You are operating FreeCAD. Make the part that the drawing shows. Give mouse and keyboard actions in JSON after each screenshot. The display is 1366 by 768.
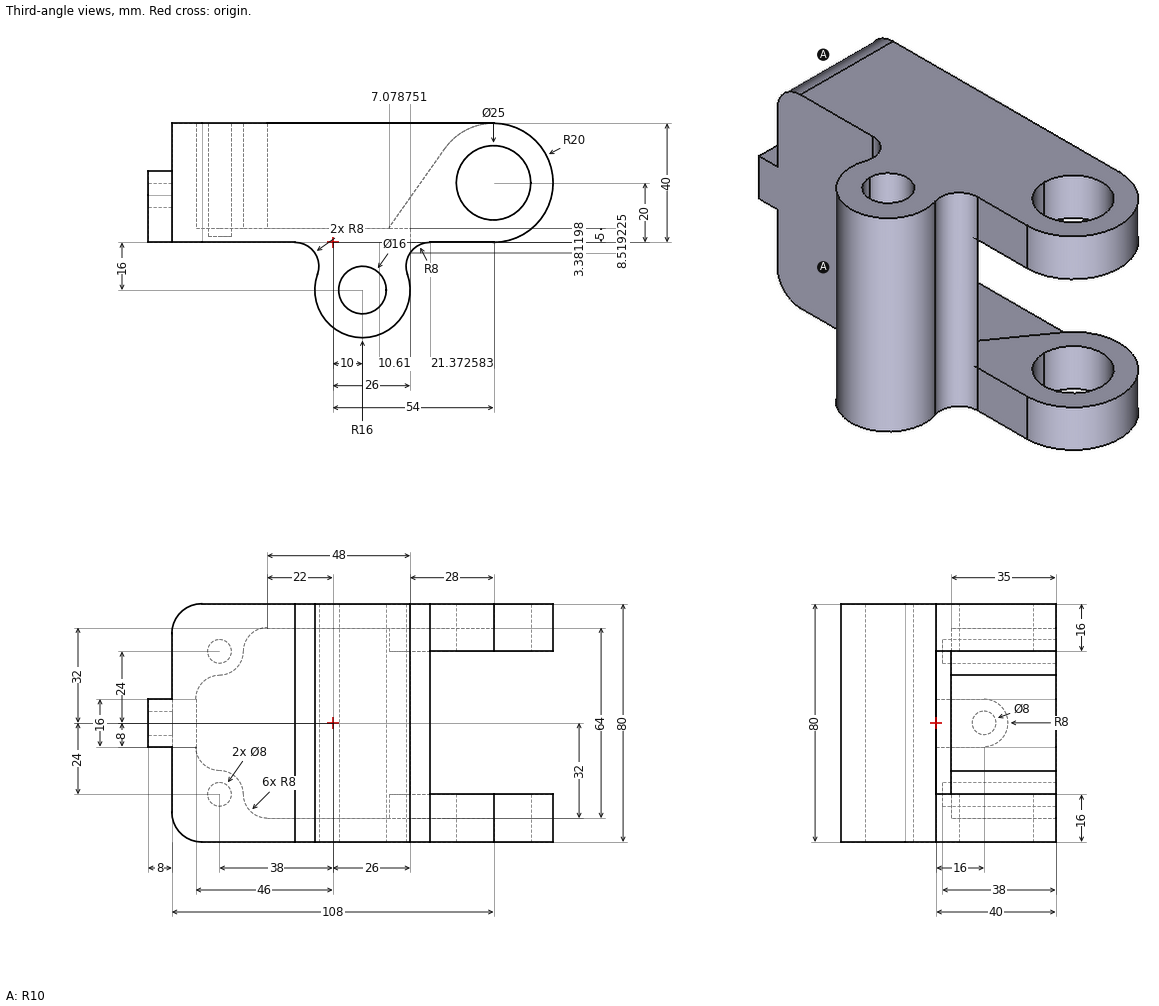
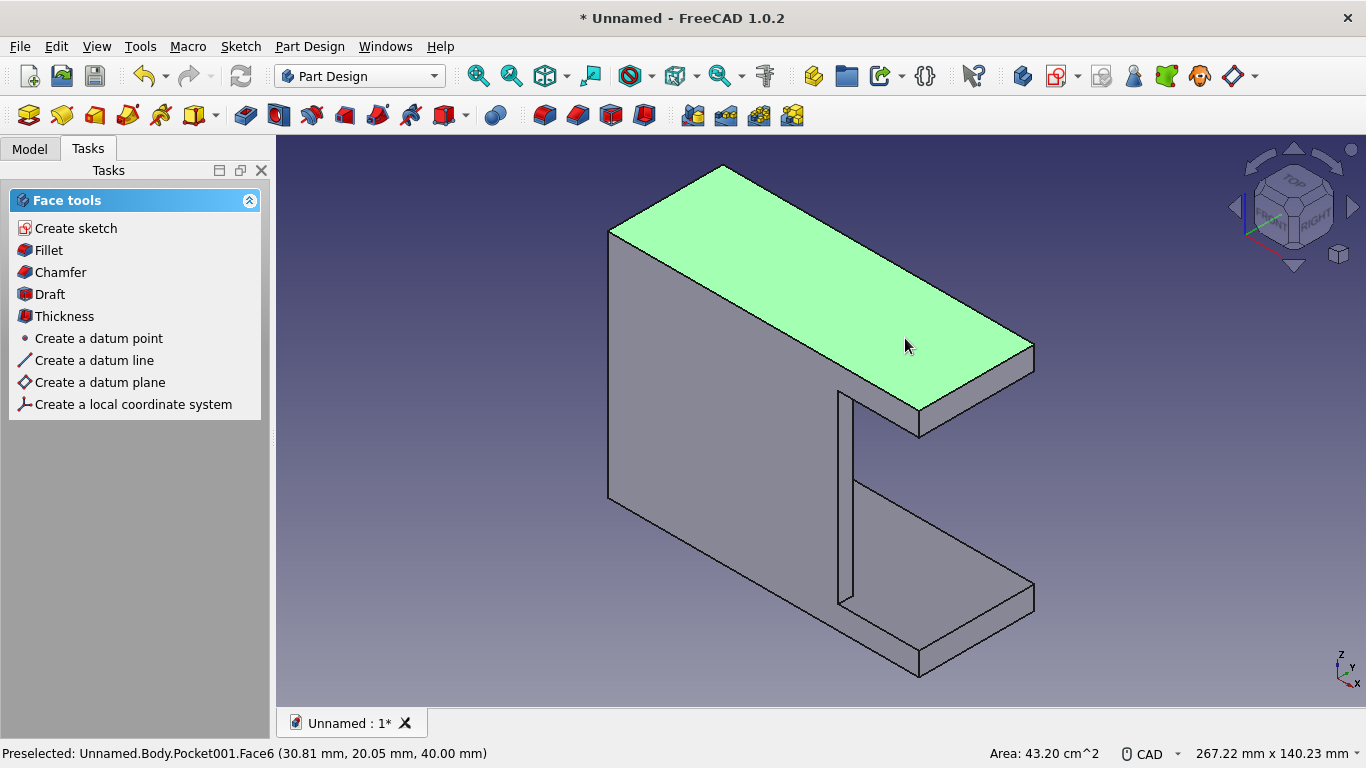
{"action": "left_click", "coordinate": [1056, 76]}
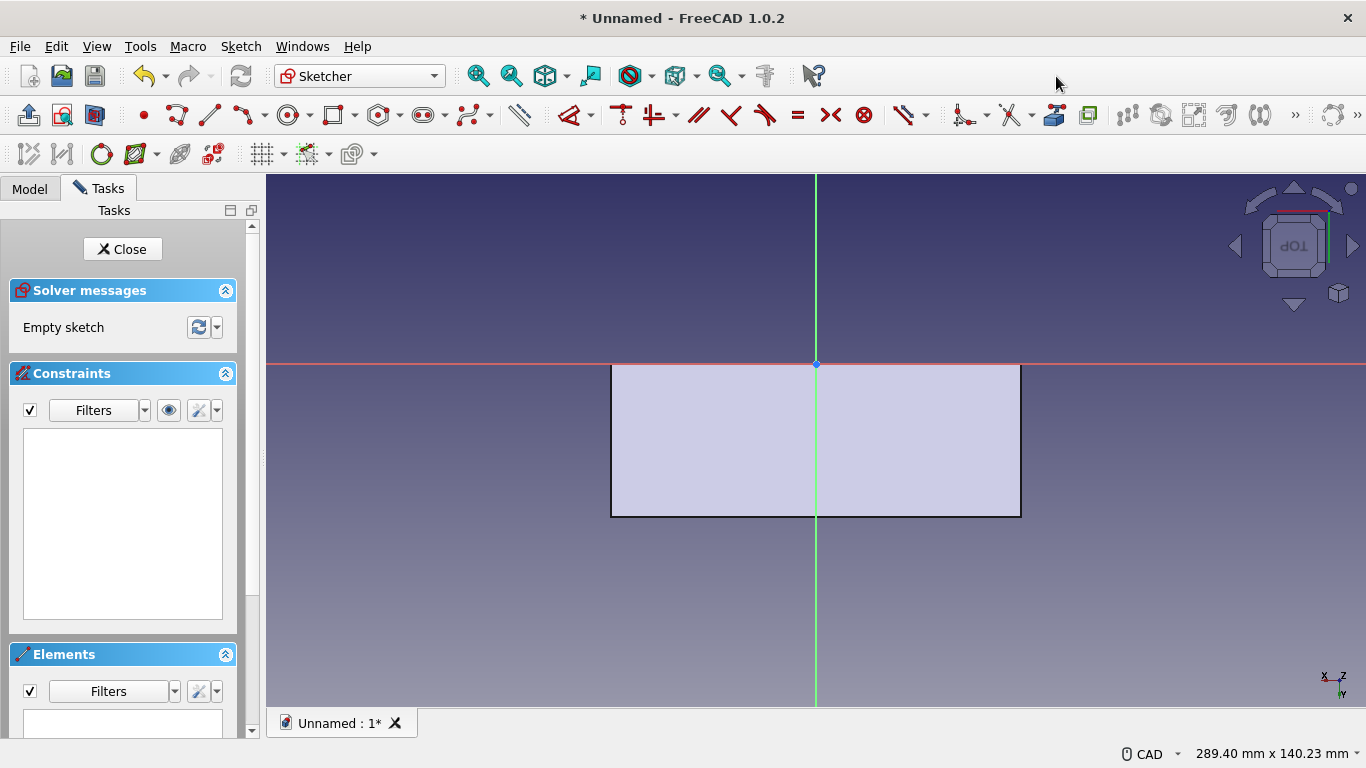
{"action": "scroll", "coordinate": [796, 224], "scroll_direction": "up", "scroll_amount": 5}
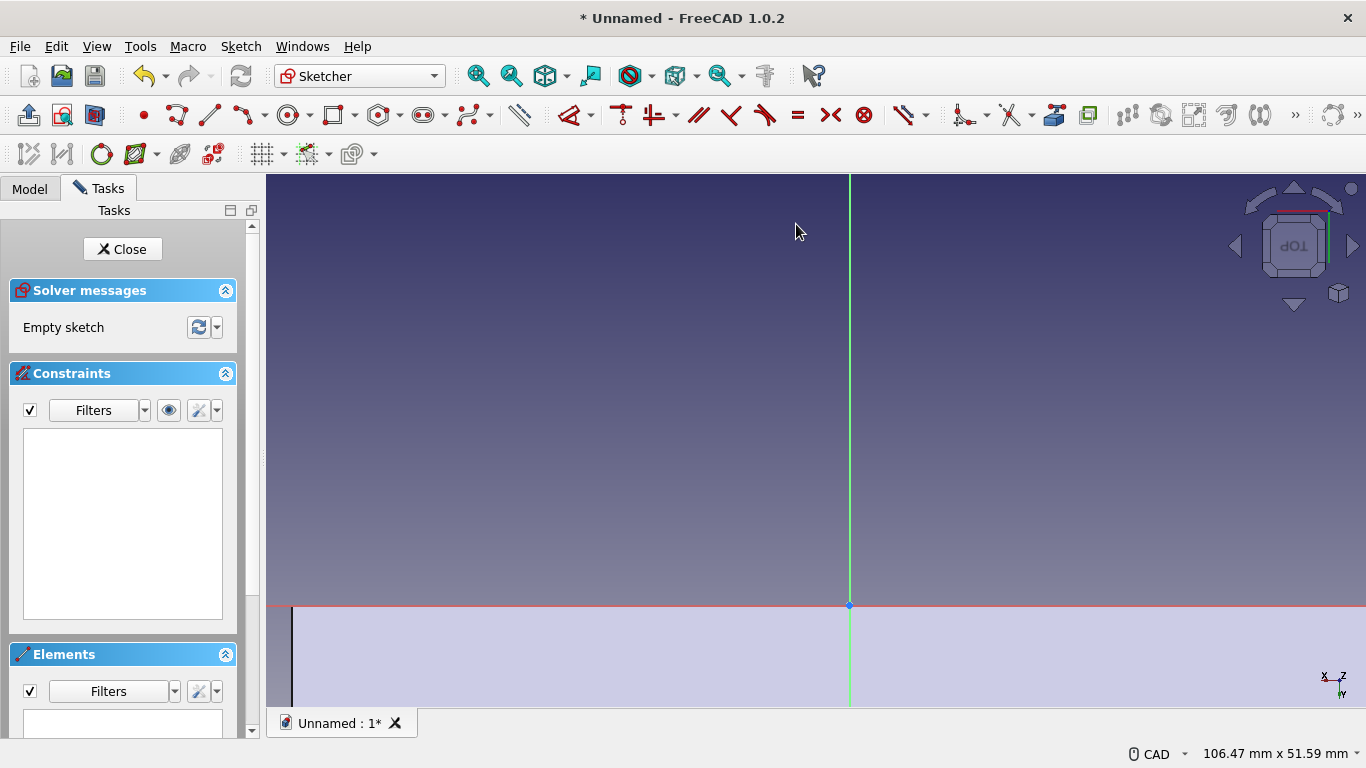
{"action": "left_click", "coordinate": [210, 116]}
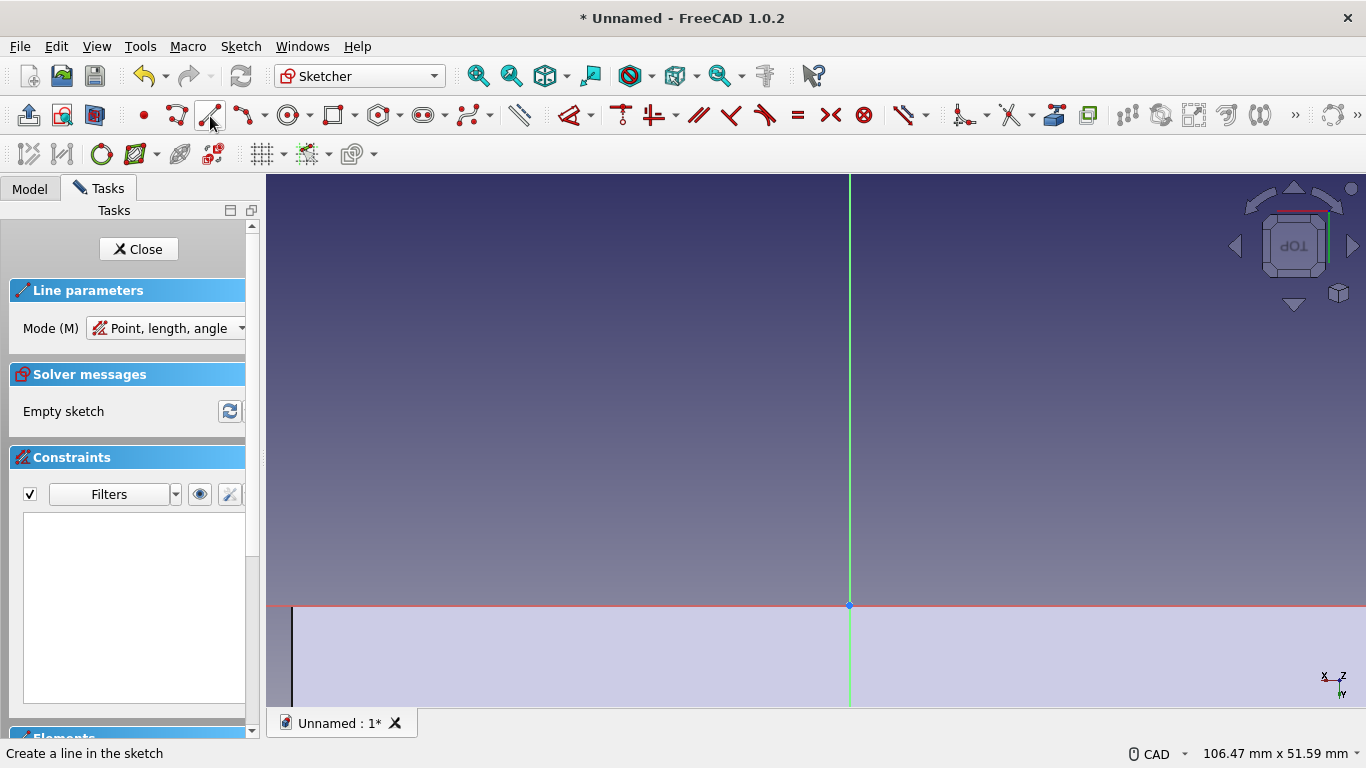
{"action": "left_click", "coordinate": [512, 606]}
{"action": "left_click", "coordinate": [980, 597]}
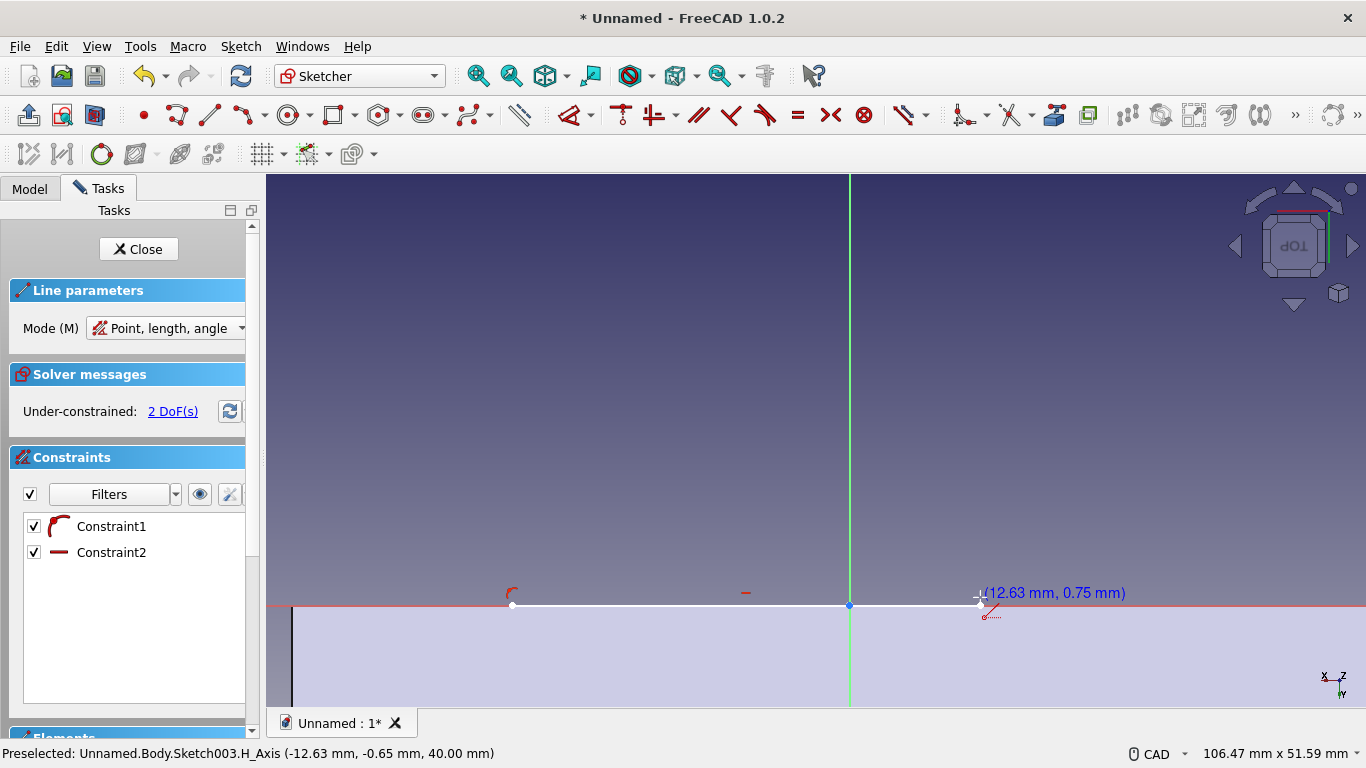
{"action": "key", "text": "g 3 a"}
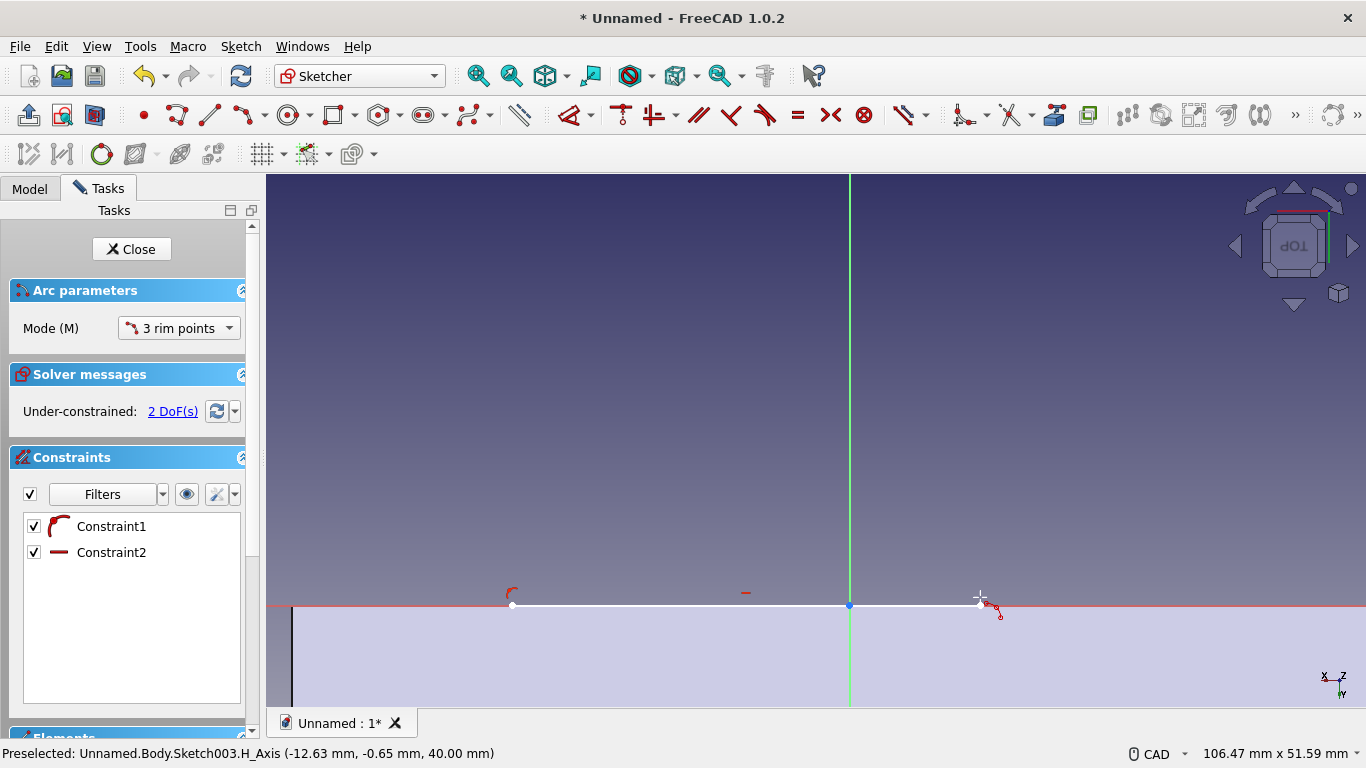
{"action": "left_click", "coordinate": [980, 606]}
{"action": "left_click", "coordinate": [902, 495]}
{"action": "left_click", "coordinate": [913, 571]}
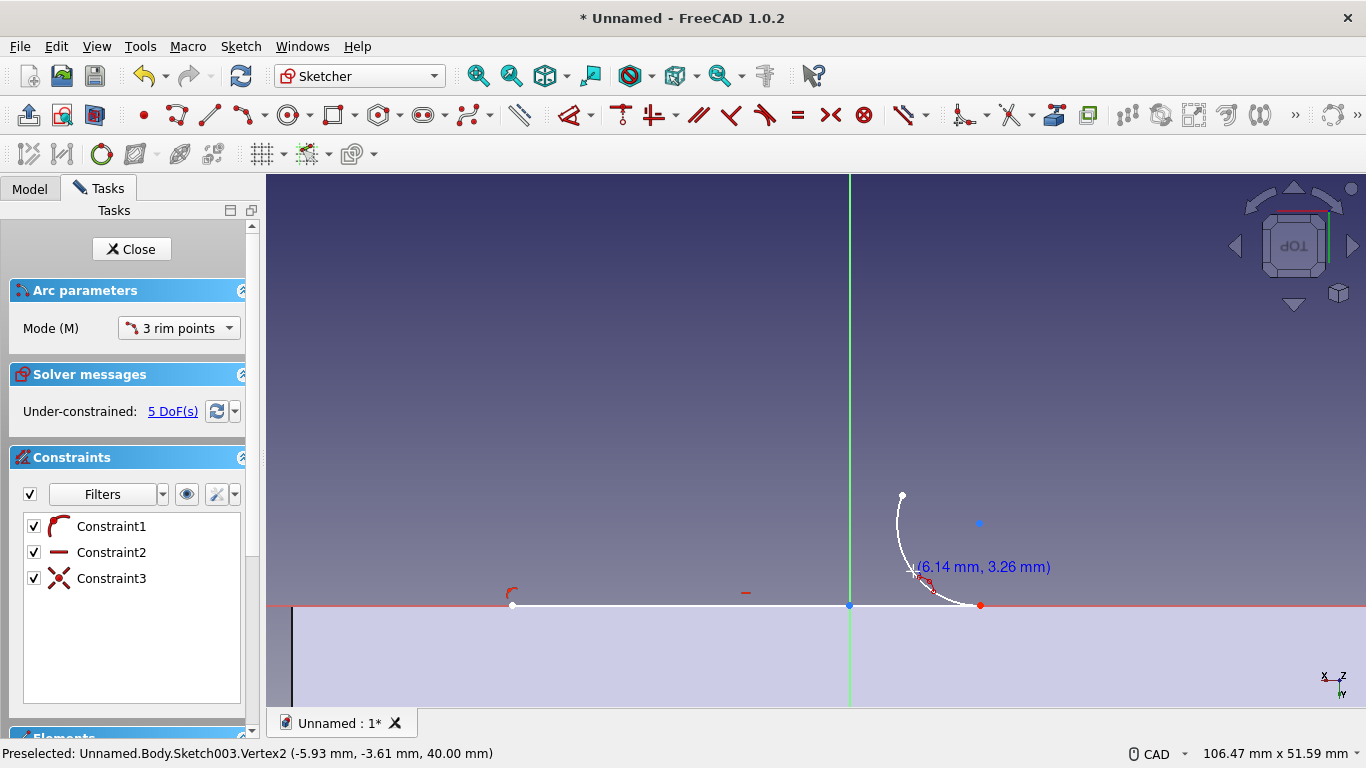
{"action": "left_click", "coordinate": [902, 496]}
{"action": "left_click", "coordinate": [590, 495]}
{"action": "left_click", "coordinate": [746, 275]}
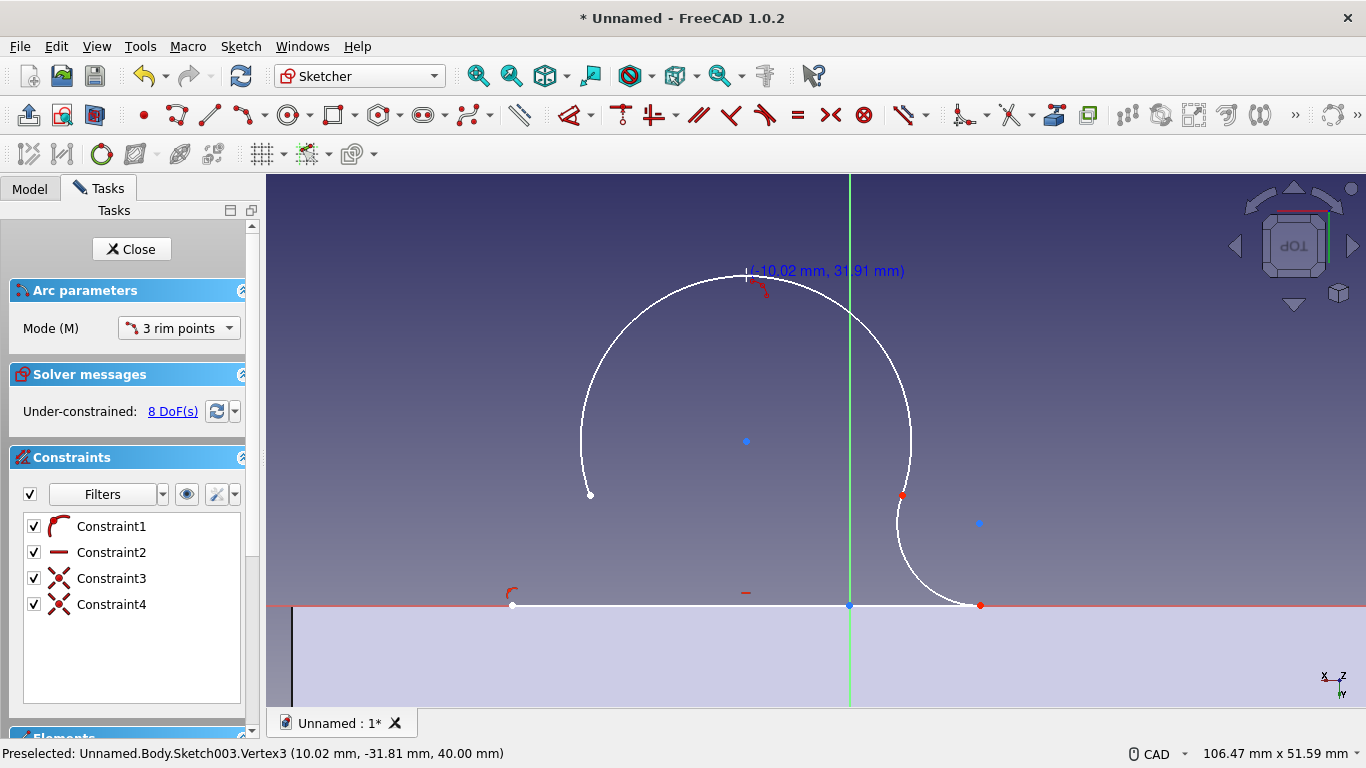
{"action": "left_click", "coordinate": [590, 496]}
{"action": "left_click", "coordinate": [512, 606]}
{"action": "left_click", "coordinate": [580, 571]}
{"action": "key", "text": "Escape"}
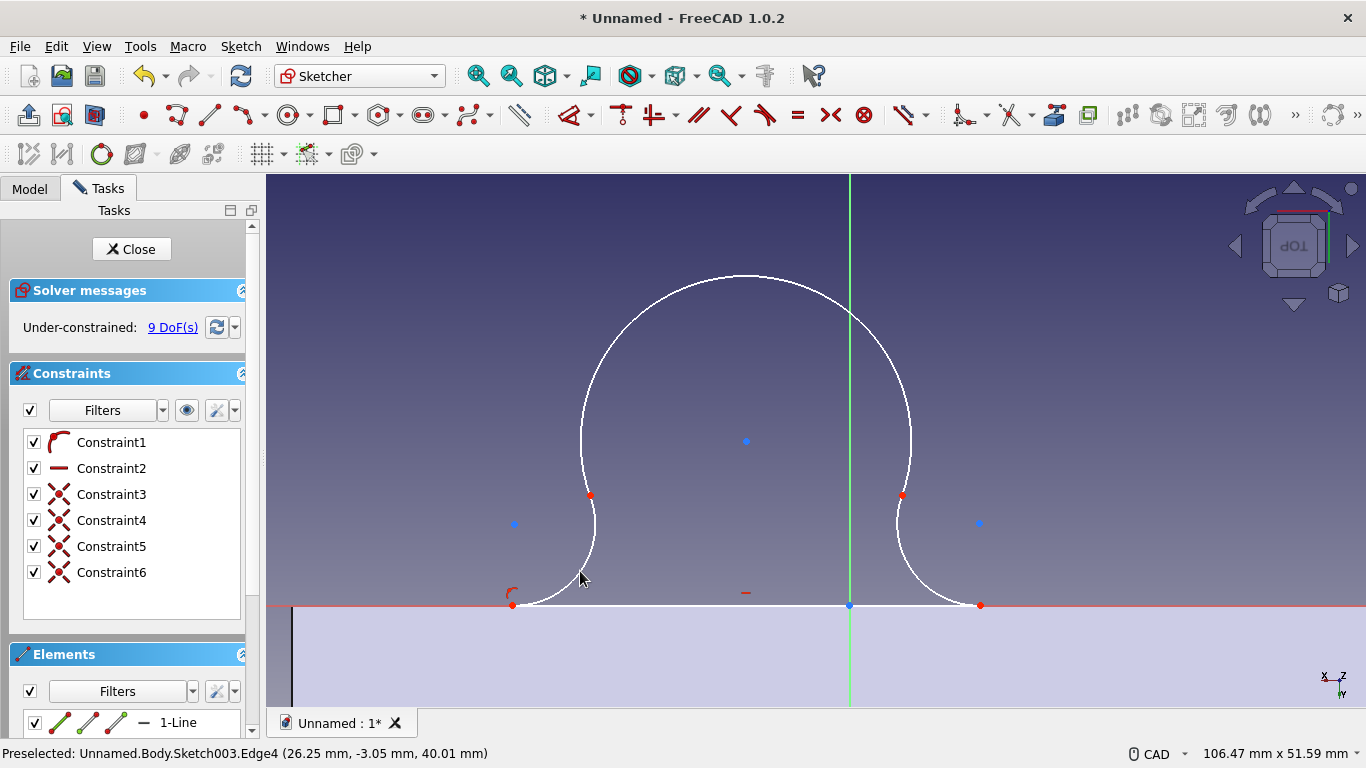
{"action": "left_click", "coordinate": [652, 606]}